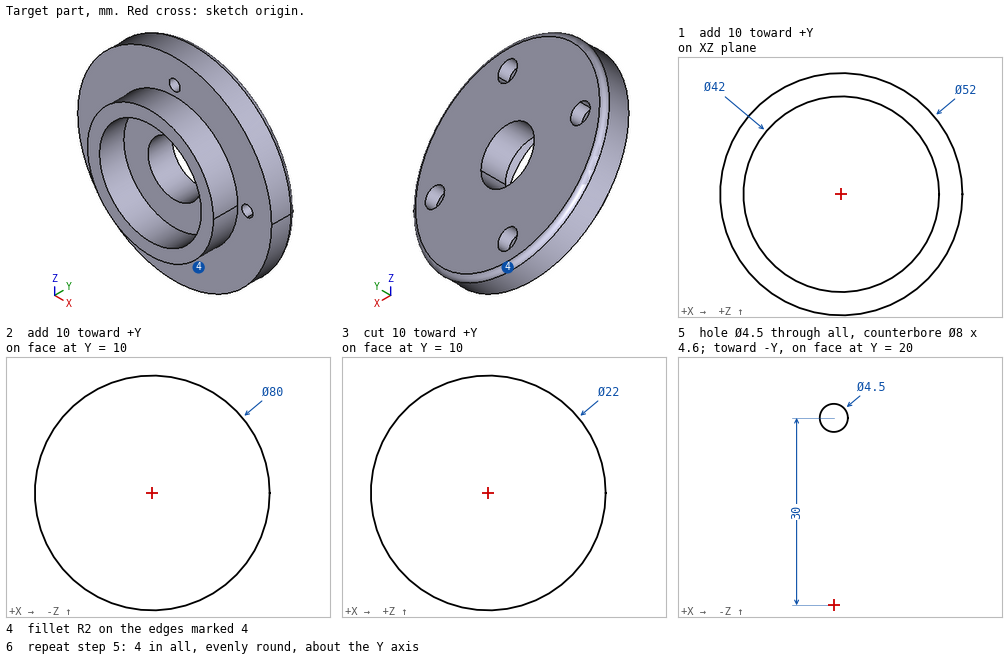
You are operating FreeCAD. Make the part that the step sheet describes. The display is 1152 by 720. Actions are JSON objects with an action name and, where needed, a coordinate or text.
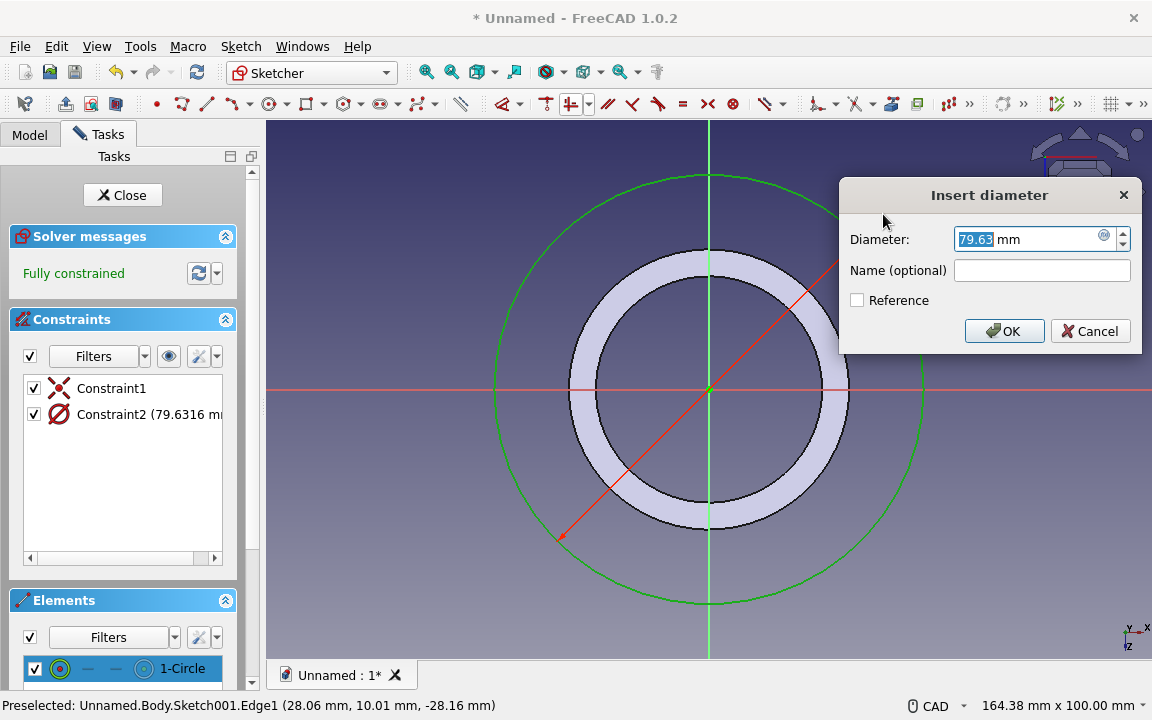
{"action": "type", "text": "80"}
{"action": "key", "text": "Return"}
{"action": "key", "text": "Escape"}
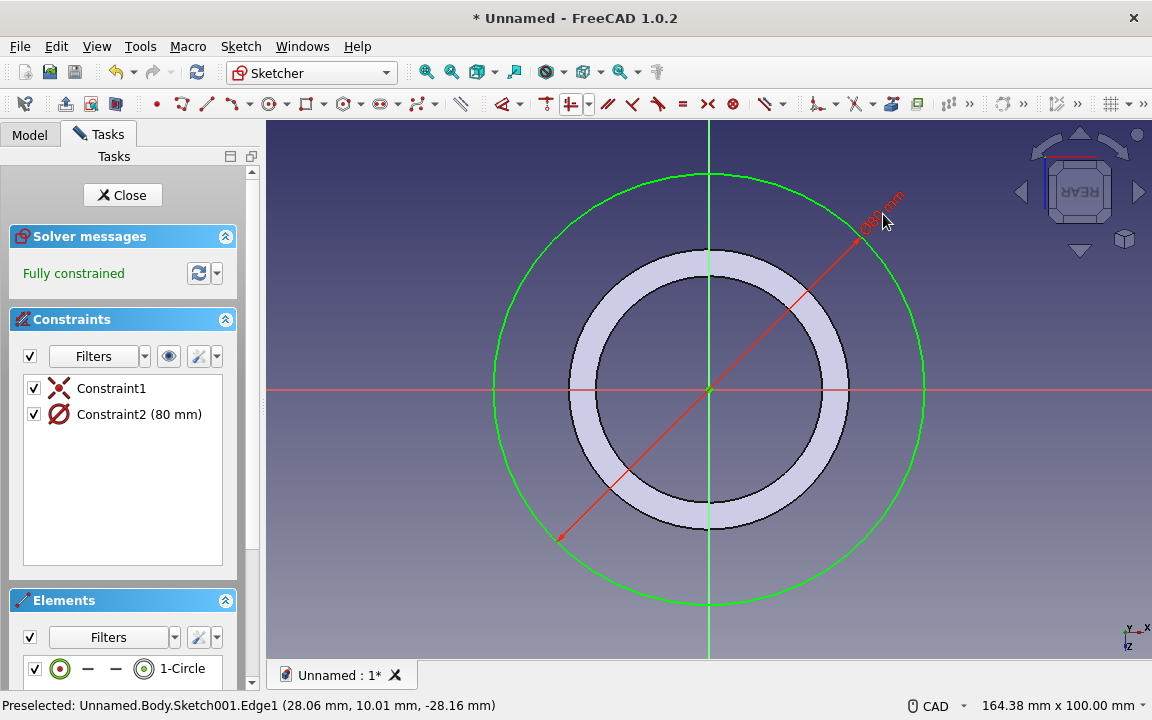
{"action": "left_click", "coordinate": [123, 195]}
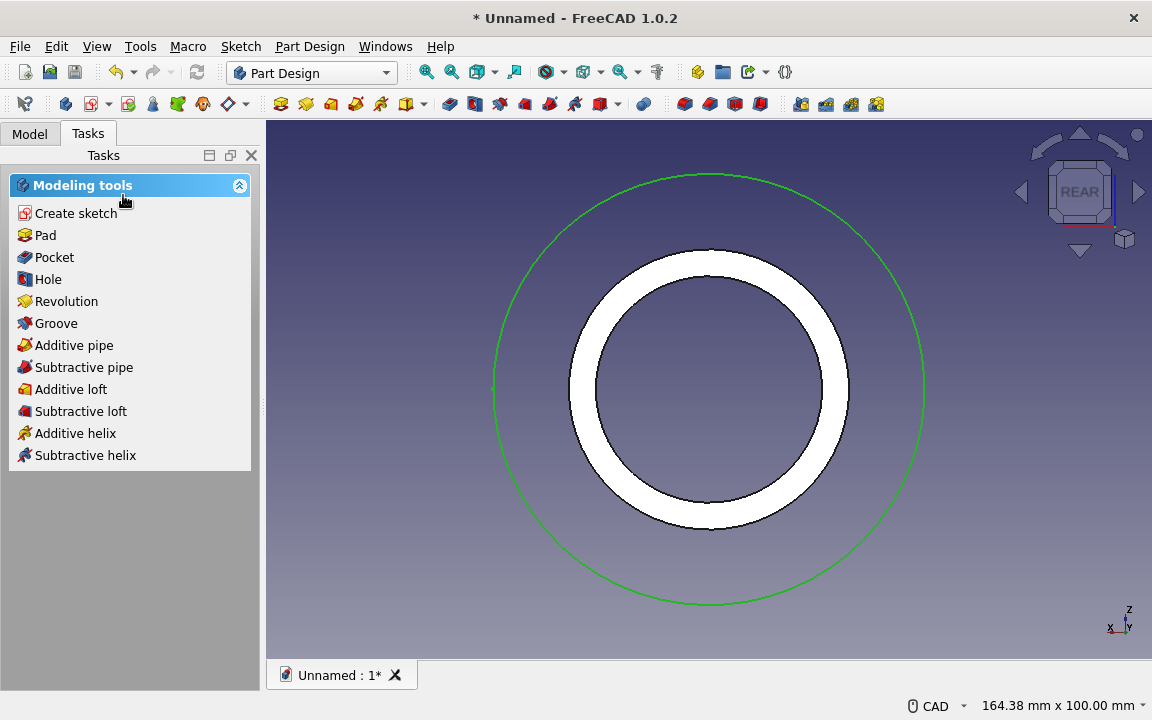
{"action": "left_click", "coordinate": [281, 104]}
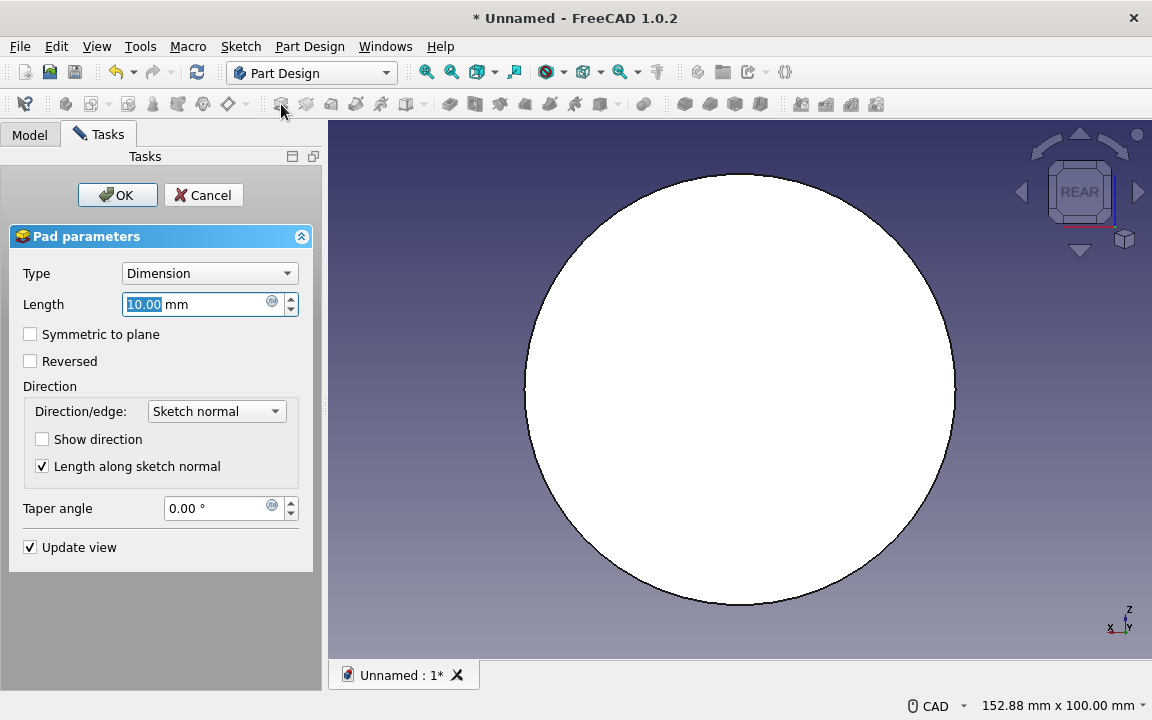
{"action": "type", "text": "10"}
{"action": "key", "text": "Tab"}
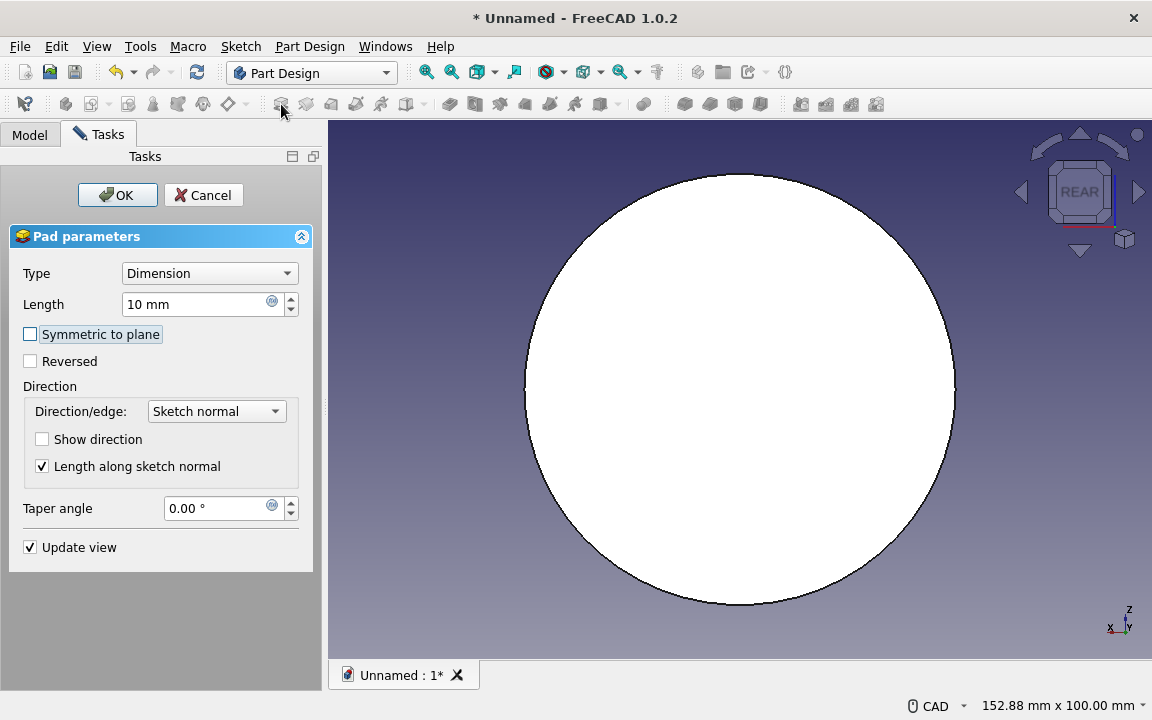
{"action": "left_click", "coordinate": [118, 195]}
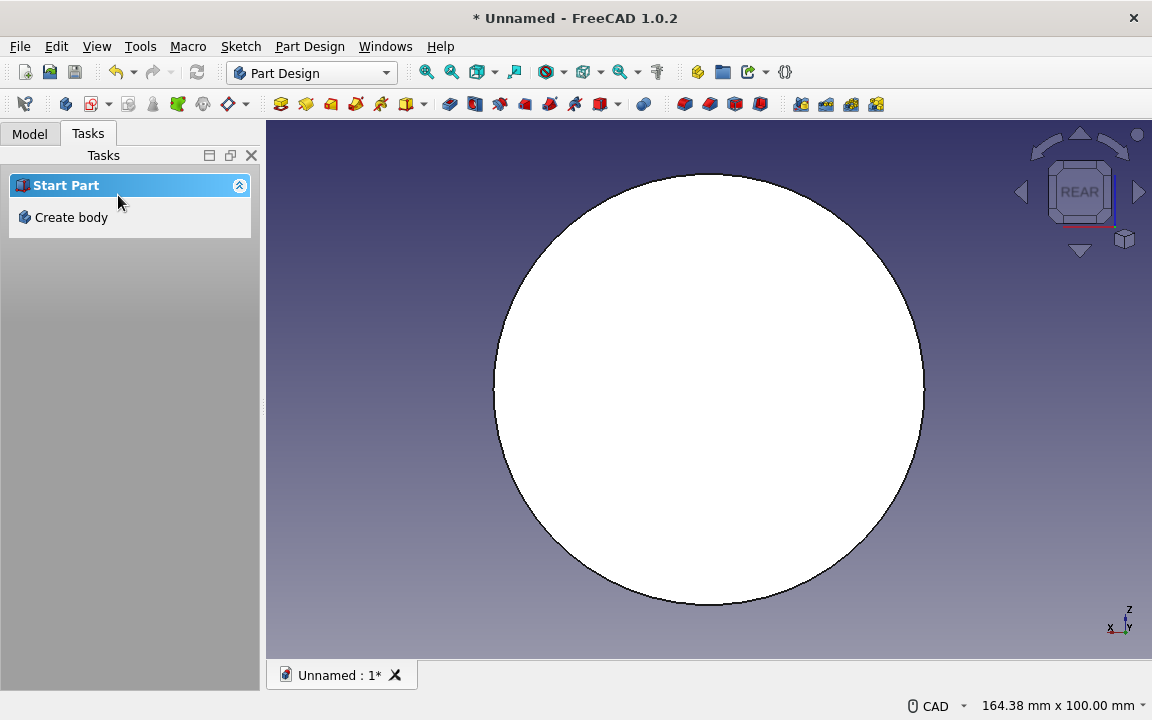
{"action": "key", "text": "0"}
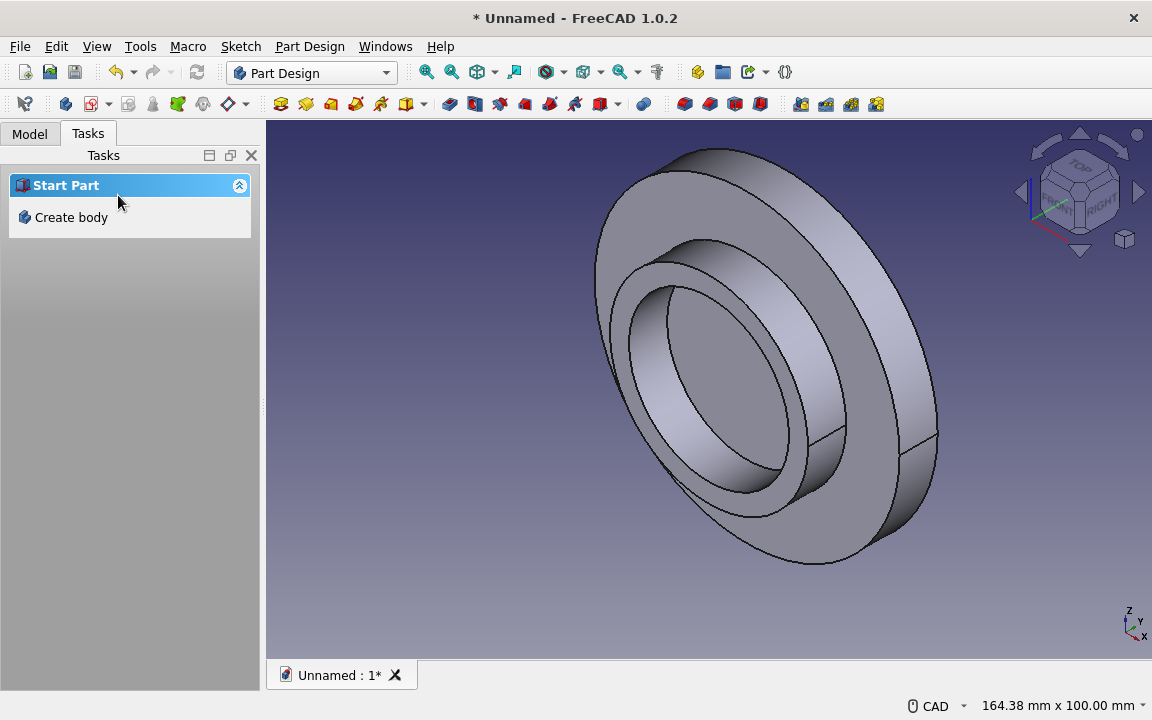
{"action": "left_click", "coordinate": [427, 72]}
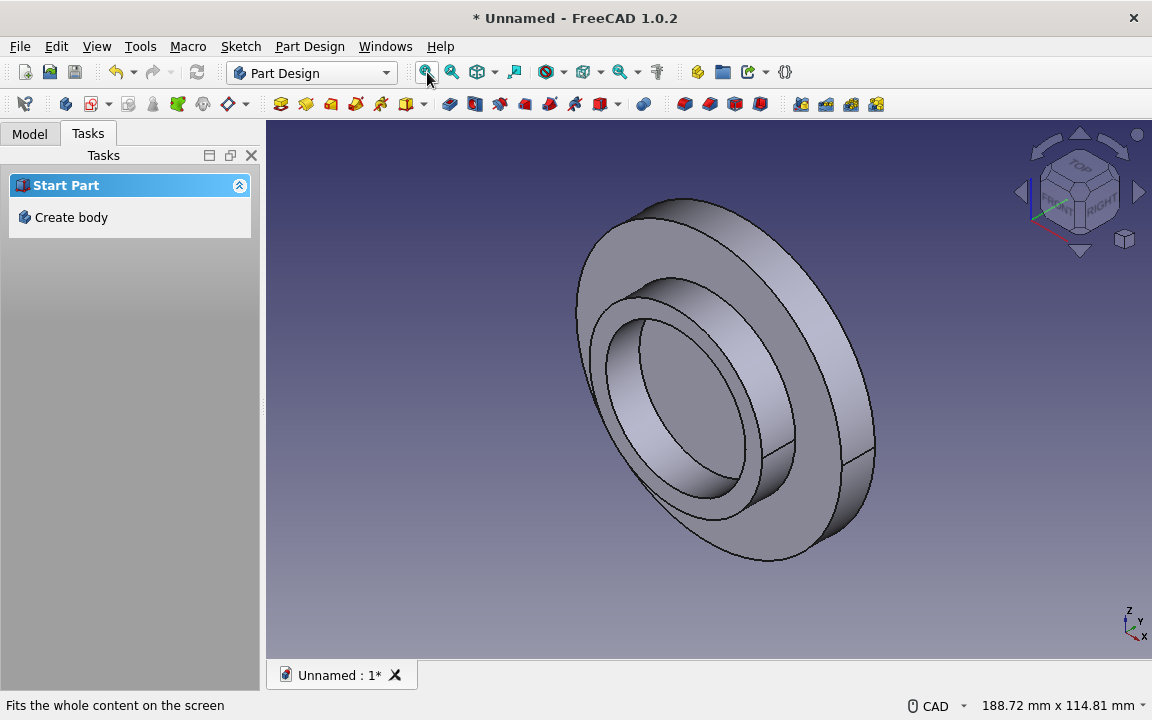
{"action": "left_click", "coordinate": [633, 257]}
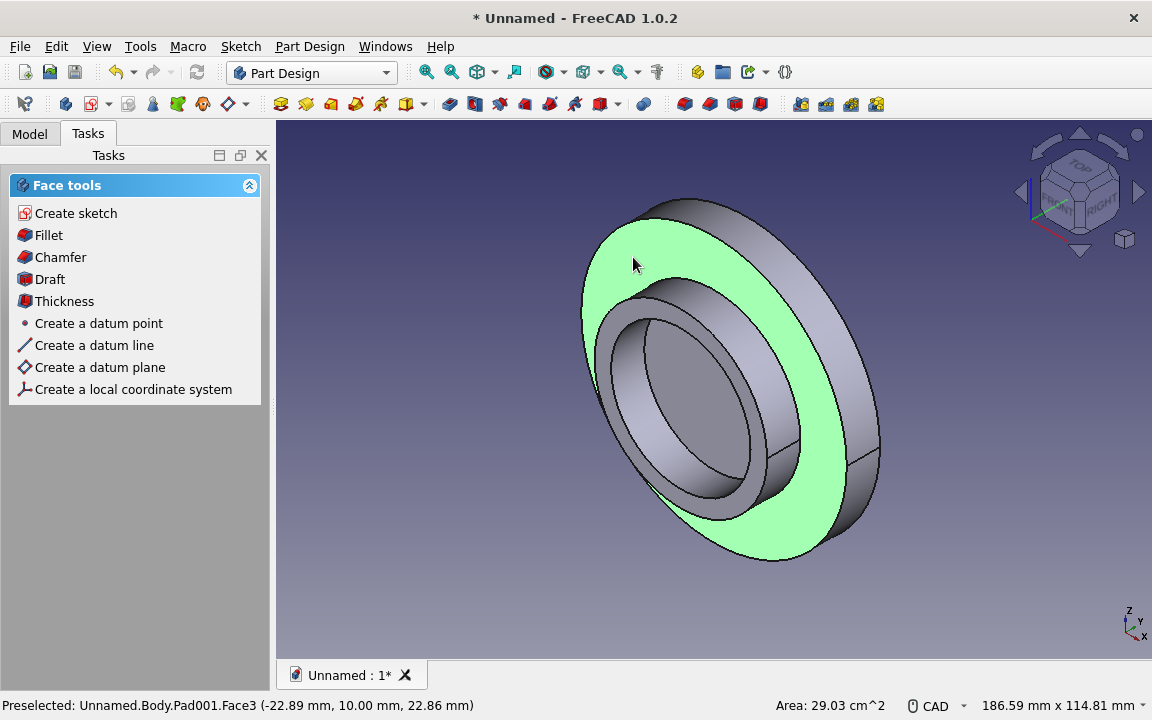
{"action": "left_click", "coordinate": [90, 104]}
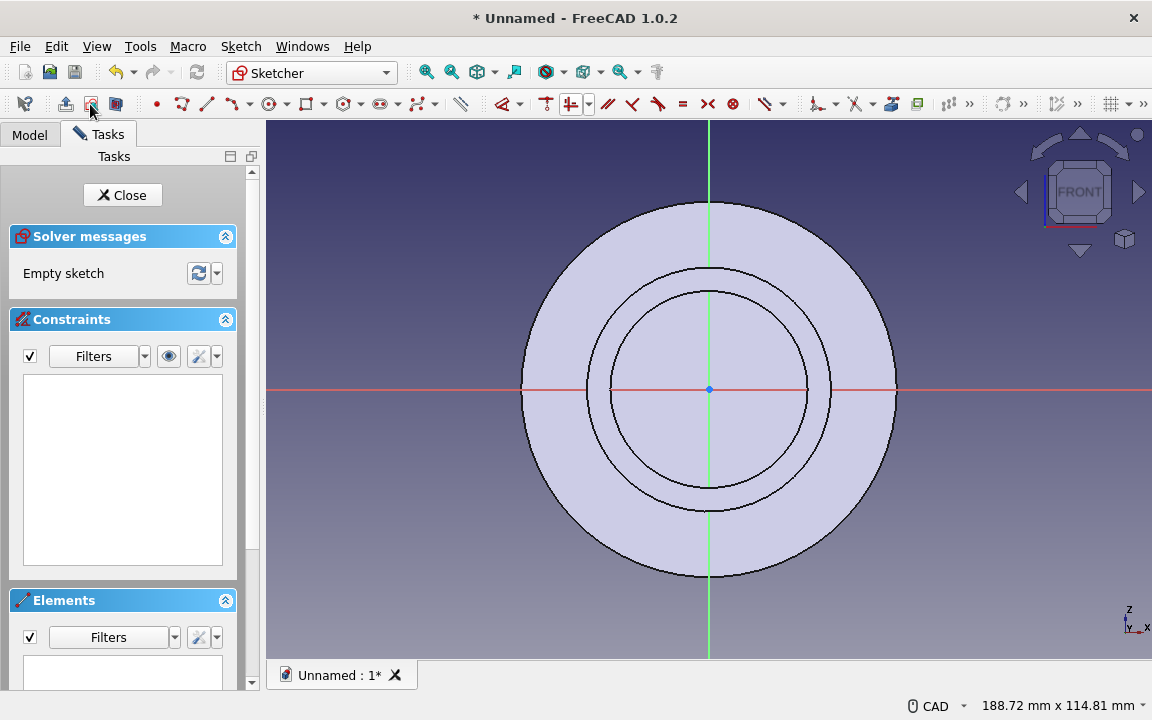
{"action": "scroll", "coordinate": [739, 390], "scroll_direction": "up", "scroll_amount": 6}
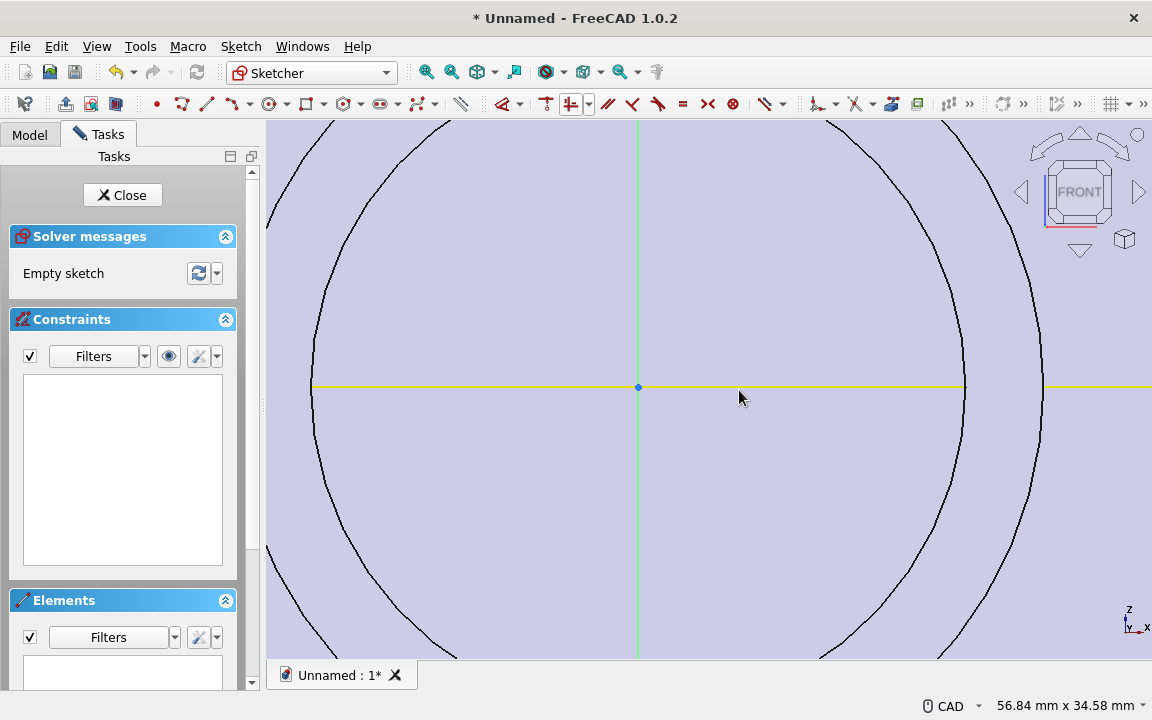
{"action": "left_click", "coordinate": [268, 104]}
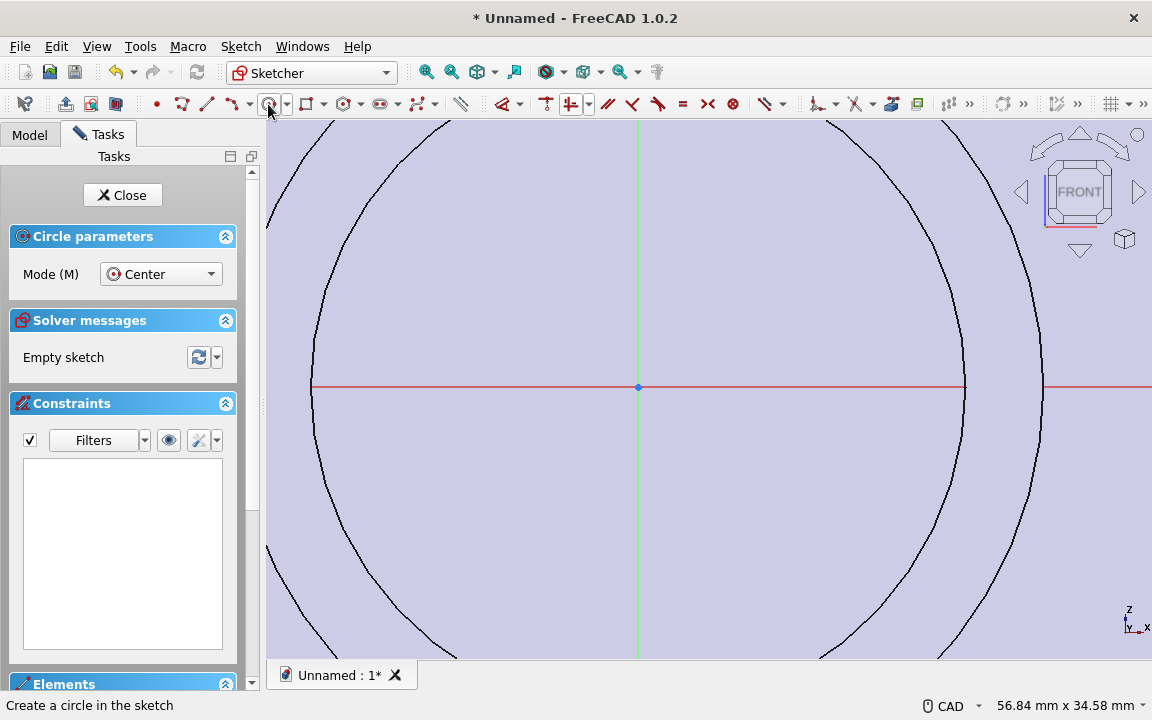
{"action": "left_click", "coordinate": [638, 387]}
{"action": "left_click", "coordinate": [759, 266]}
{"action": "key", "text": "Escape"}